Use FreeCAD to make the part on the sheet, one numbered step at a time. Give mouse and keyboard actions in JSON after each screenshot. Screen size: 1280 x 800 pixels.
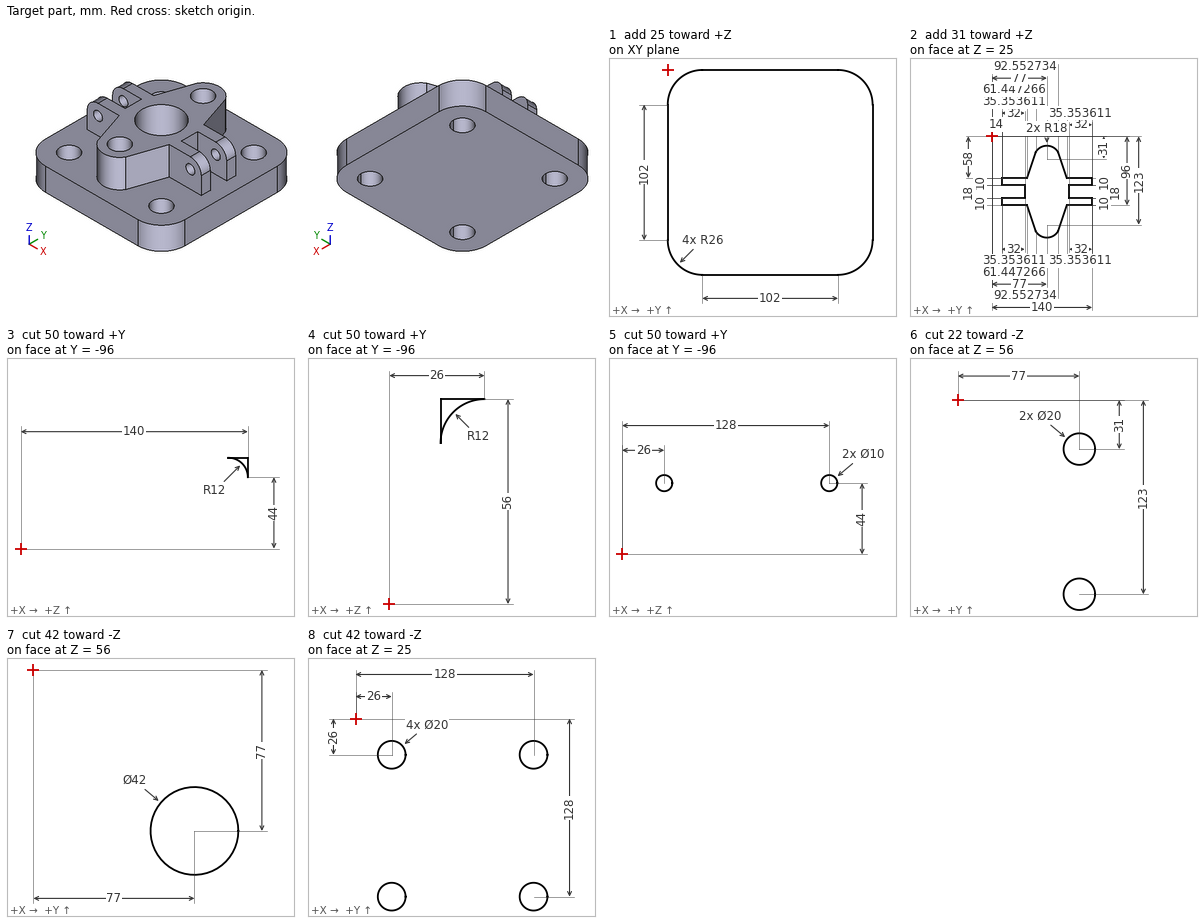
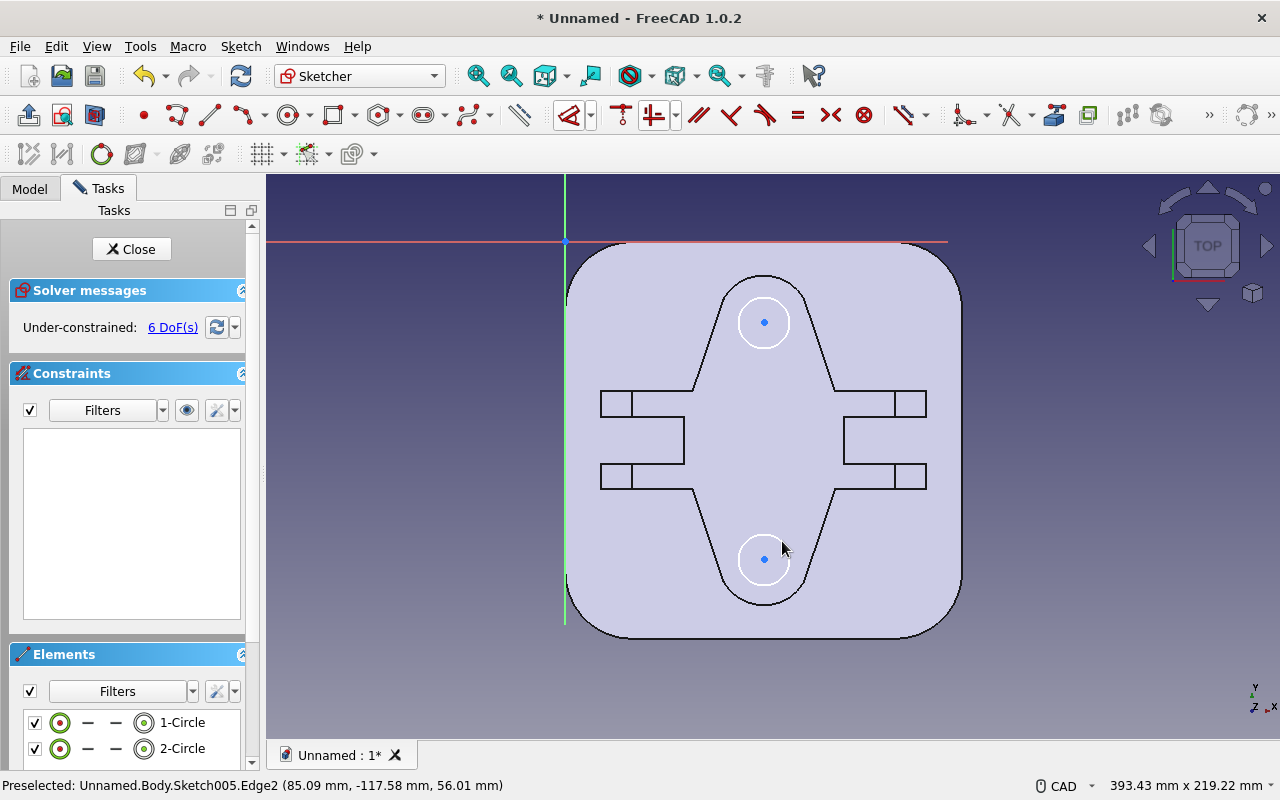
{"action": "left_click", "coordinate": [782, 305]}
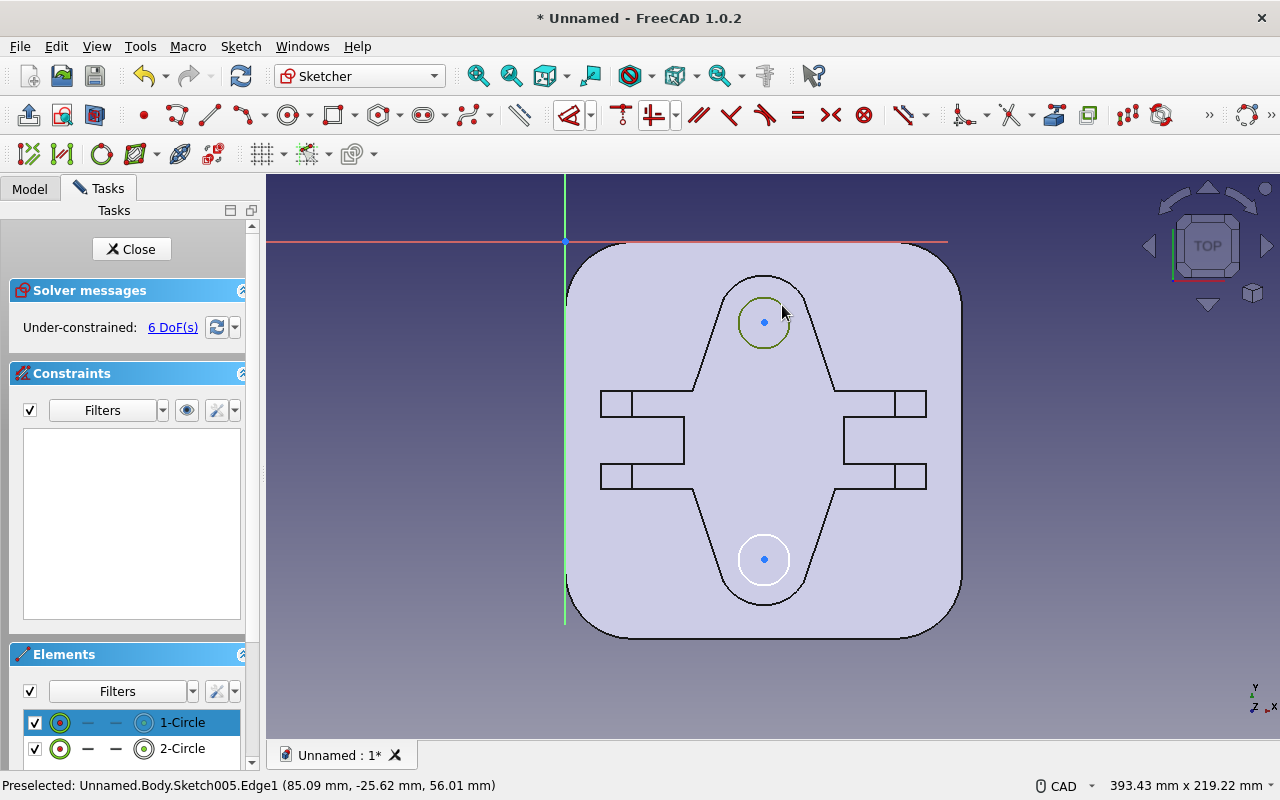
{"action": "left_click", "coordinate": [782, 542]}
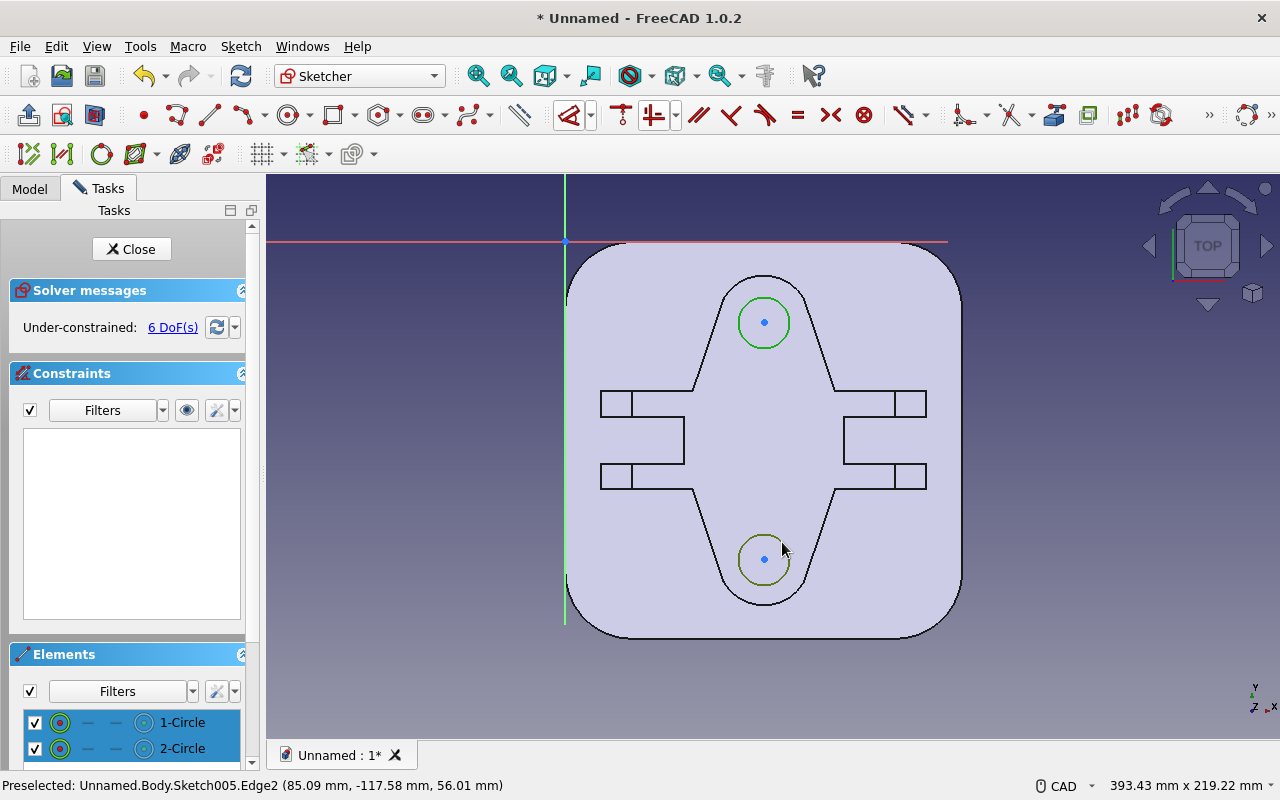
{"action": "left_click", "coordinate": [798, 116]}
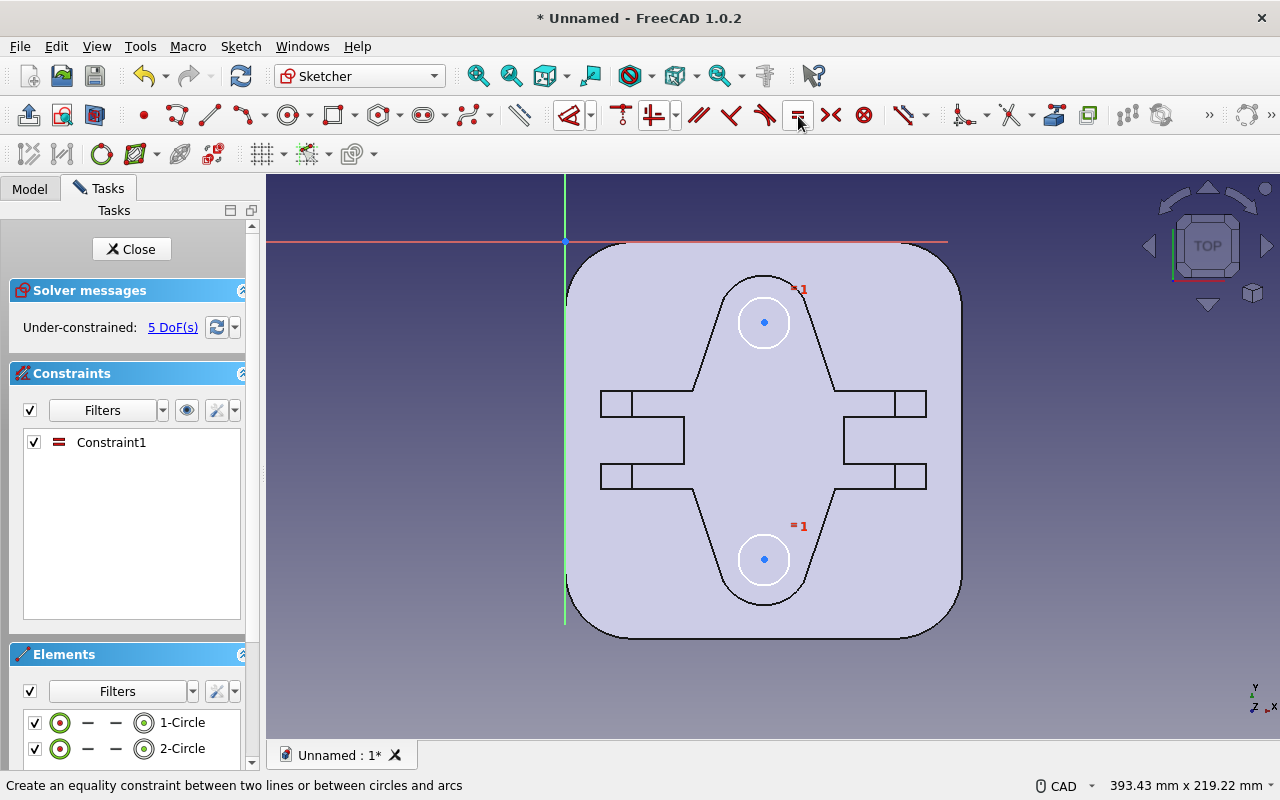
{"action": "left_click", "coordinate": [764, 323]}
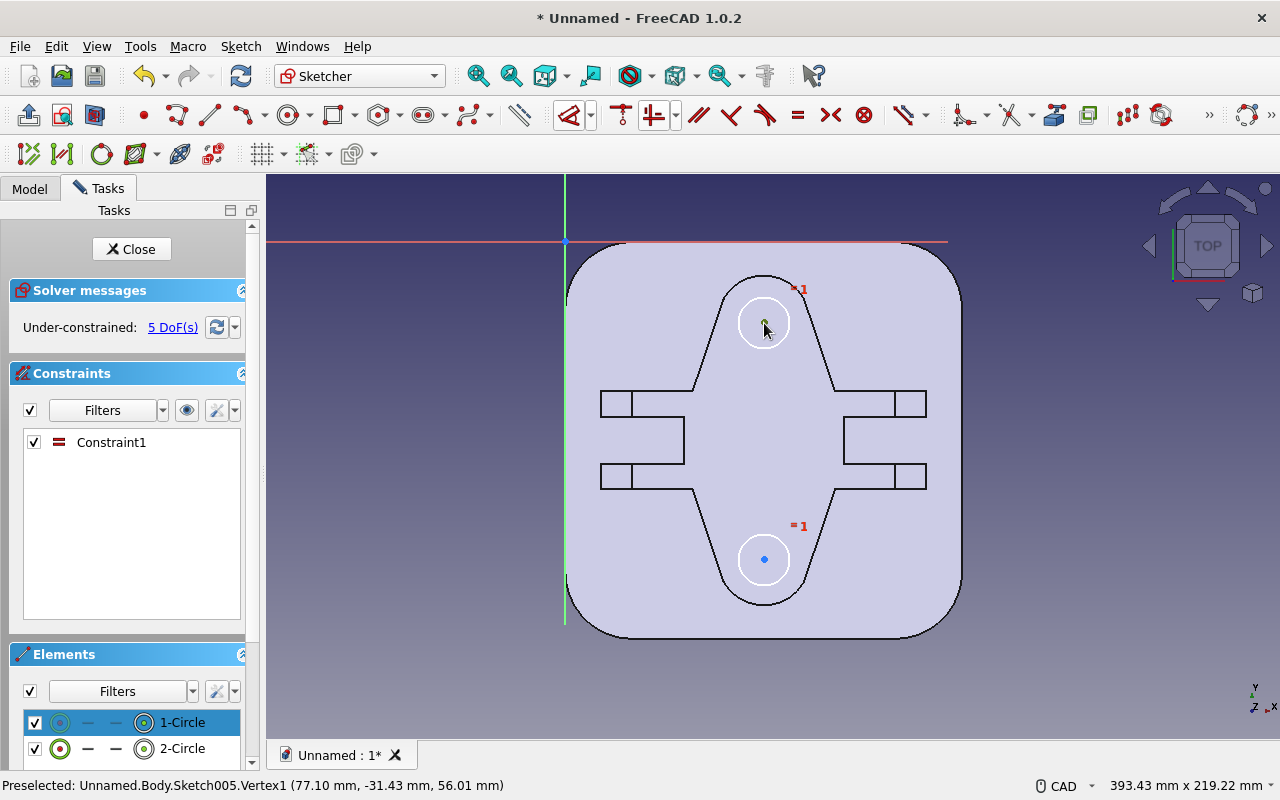
{"action": "left_click", "coordinate": [764, 560]}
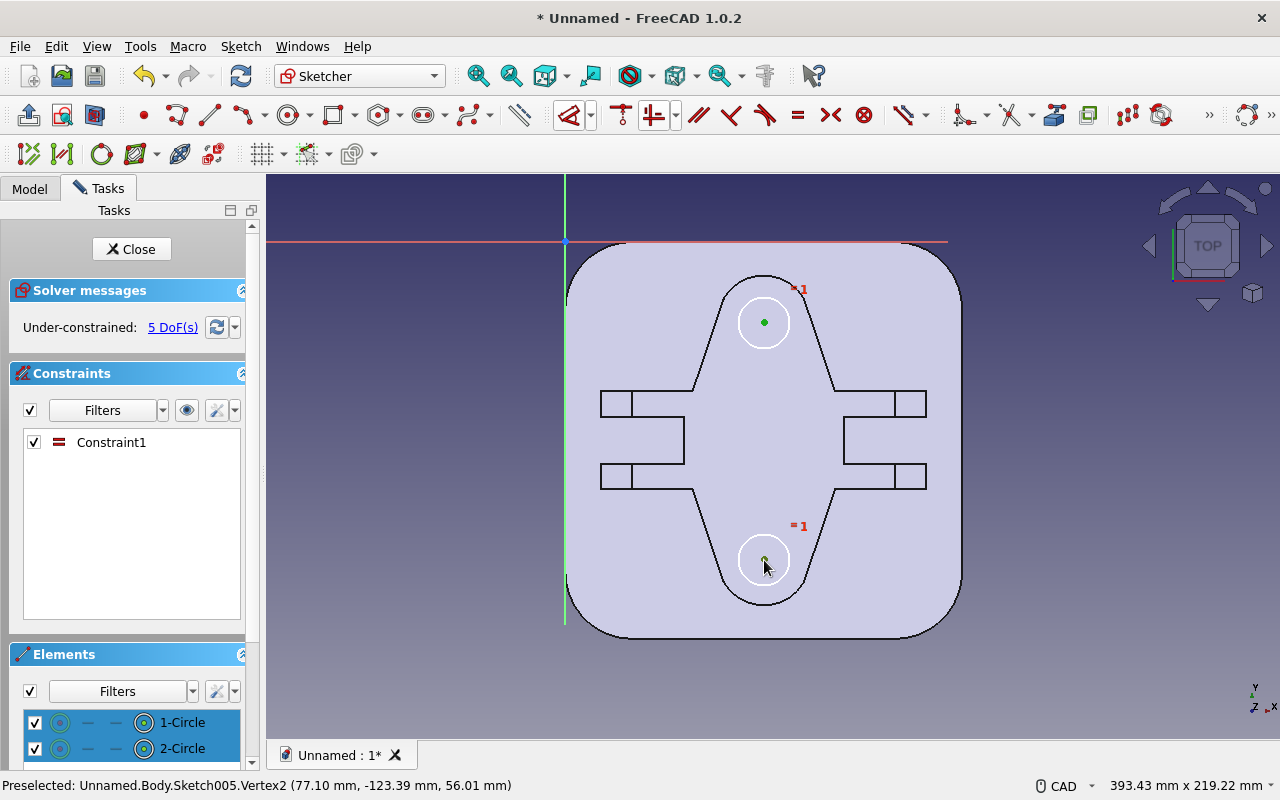
{"action": "left_click", "coordinate": [676, 116]}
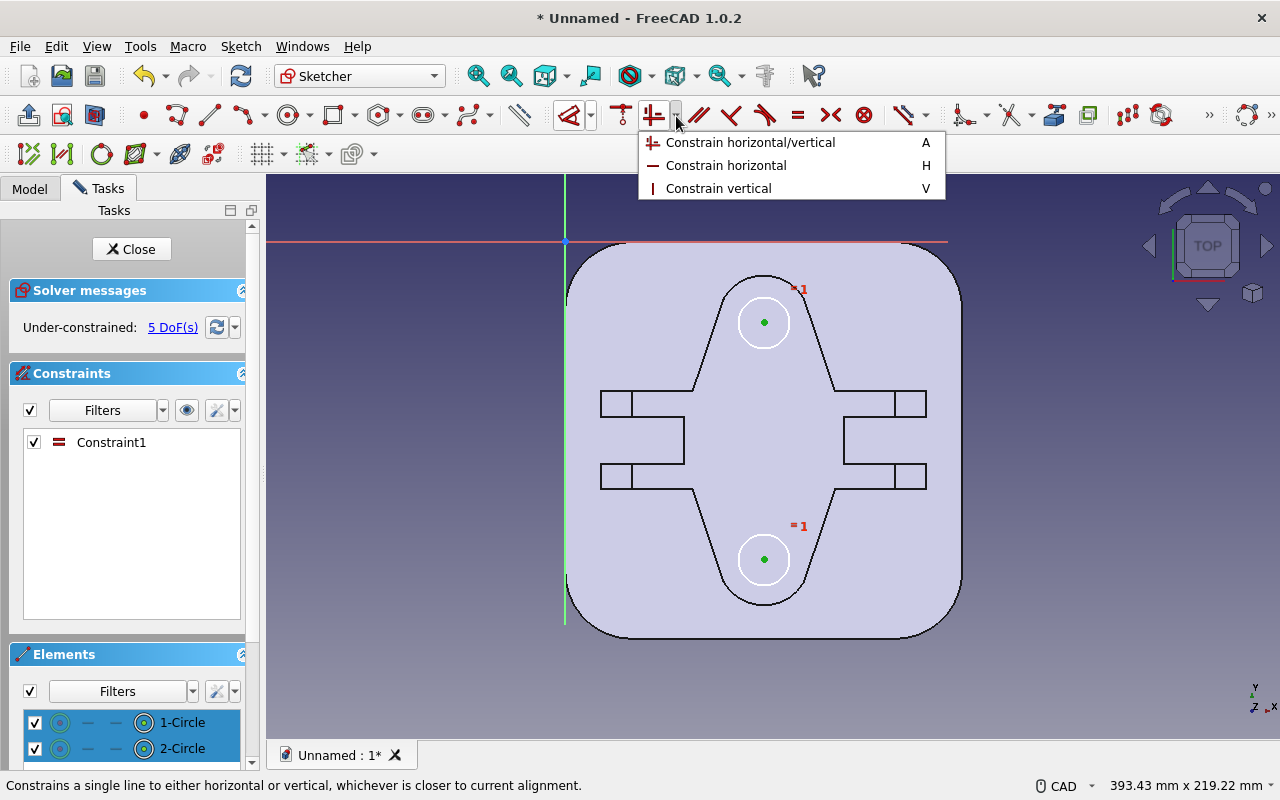
{"action": "left_click", "coordinate": [792, 188]}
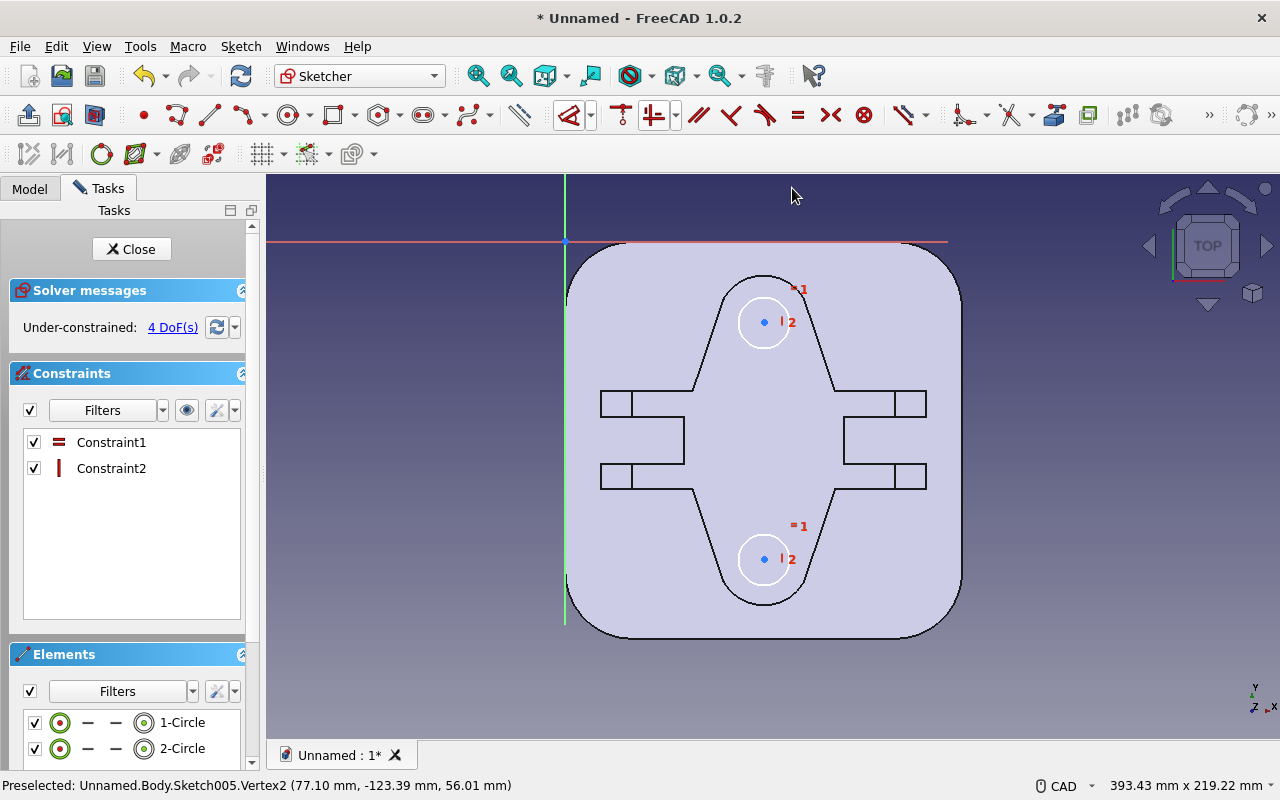
{"action": "left_click", "coordinate": [782, 305]}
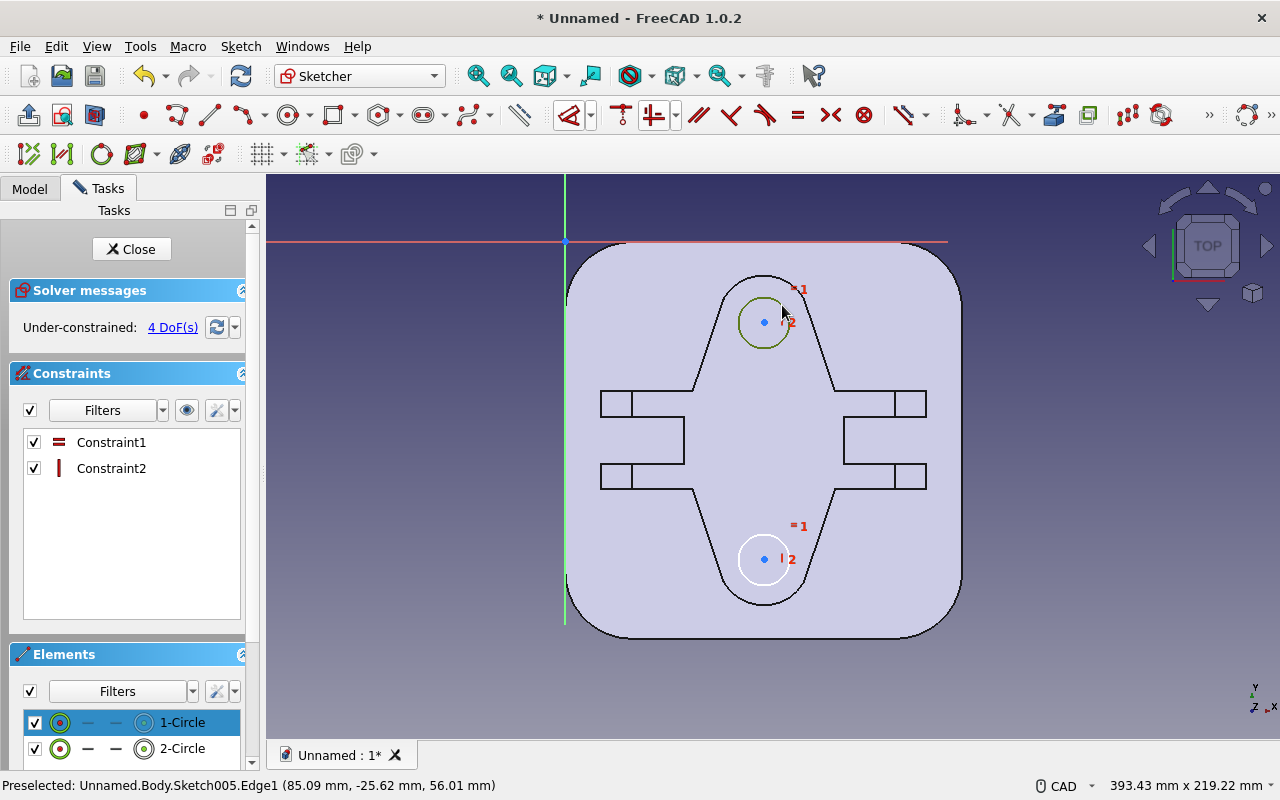
{"action": "key", "text": "k o"}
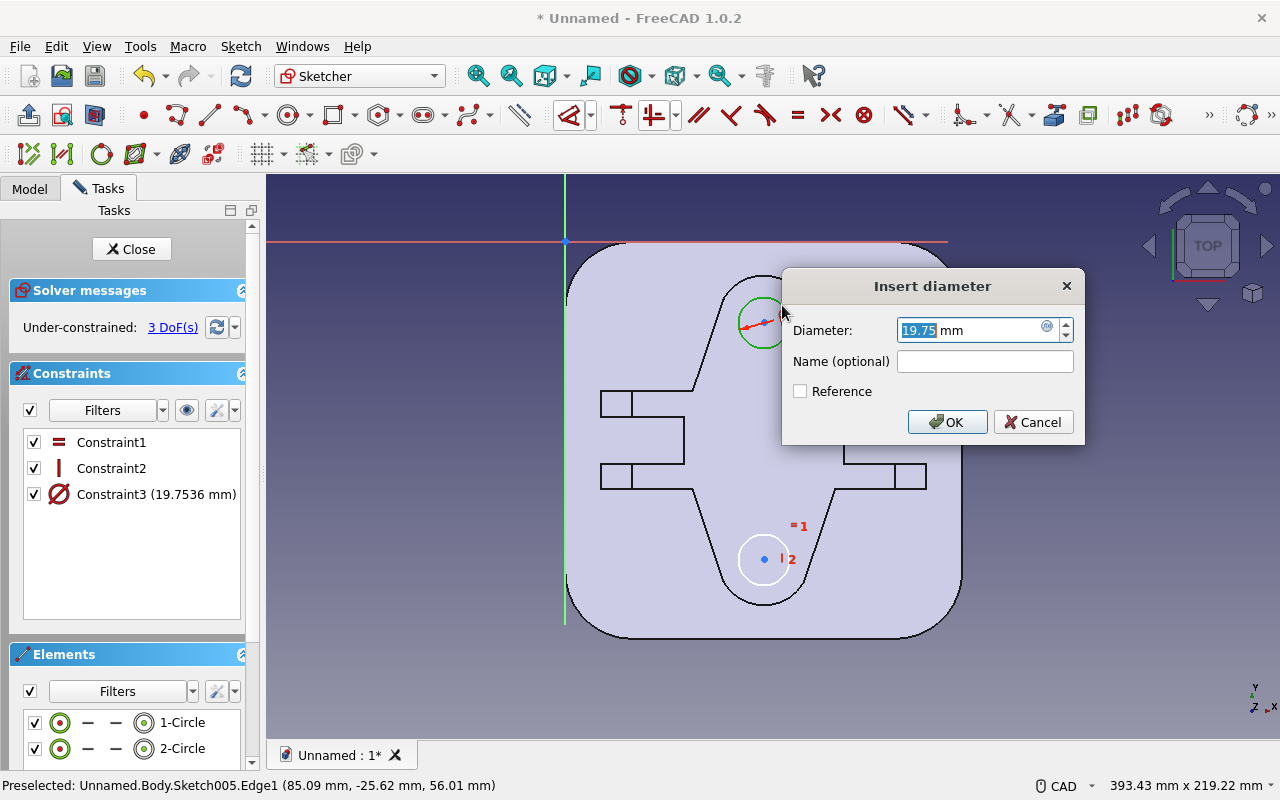
{"action": "type", "text": "20"}
{"action": "key", "text": "Return"}